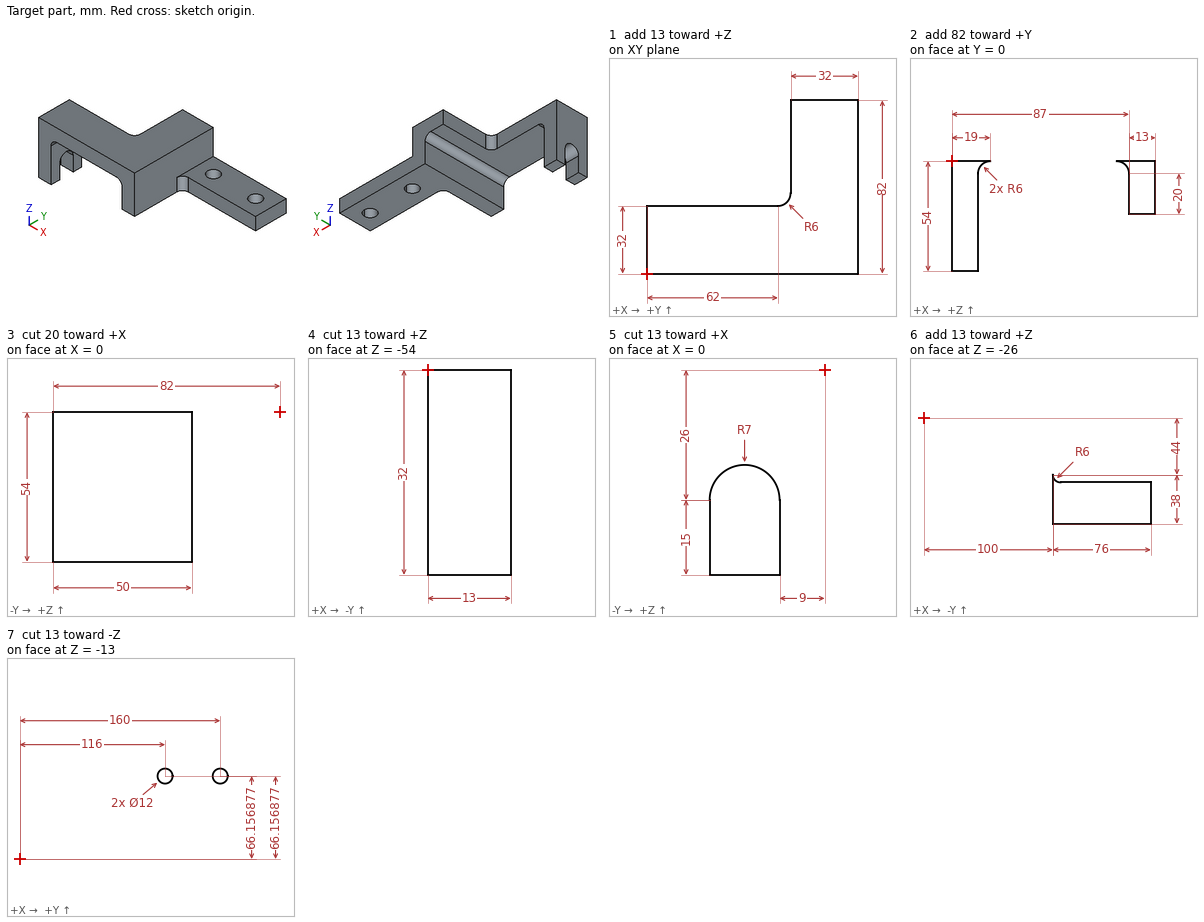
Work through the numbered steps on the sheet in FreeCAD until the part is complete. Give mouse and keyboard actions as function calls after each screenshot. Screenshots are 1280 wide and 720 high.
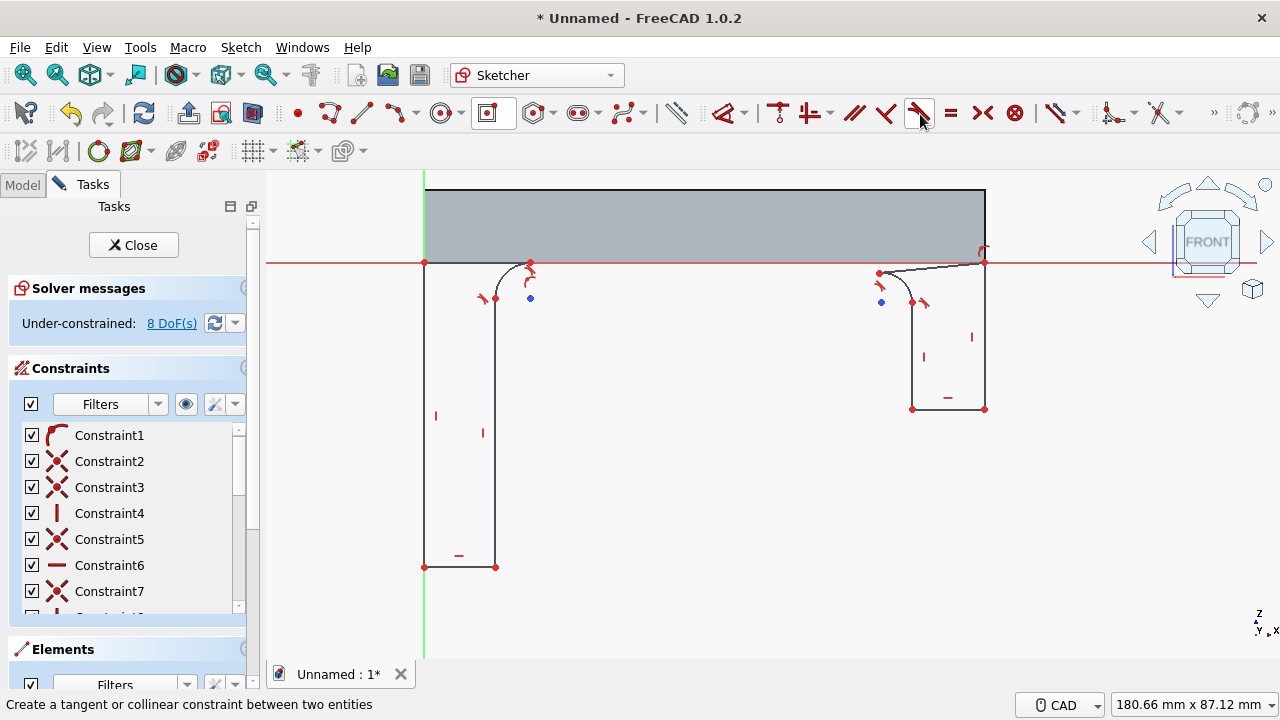
click(953, 266)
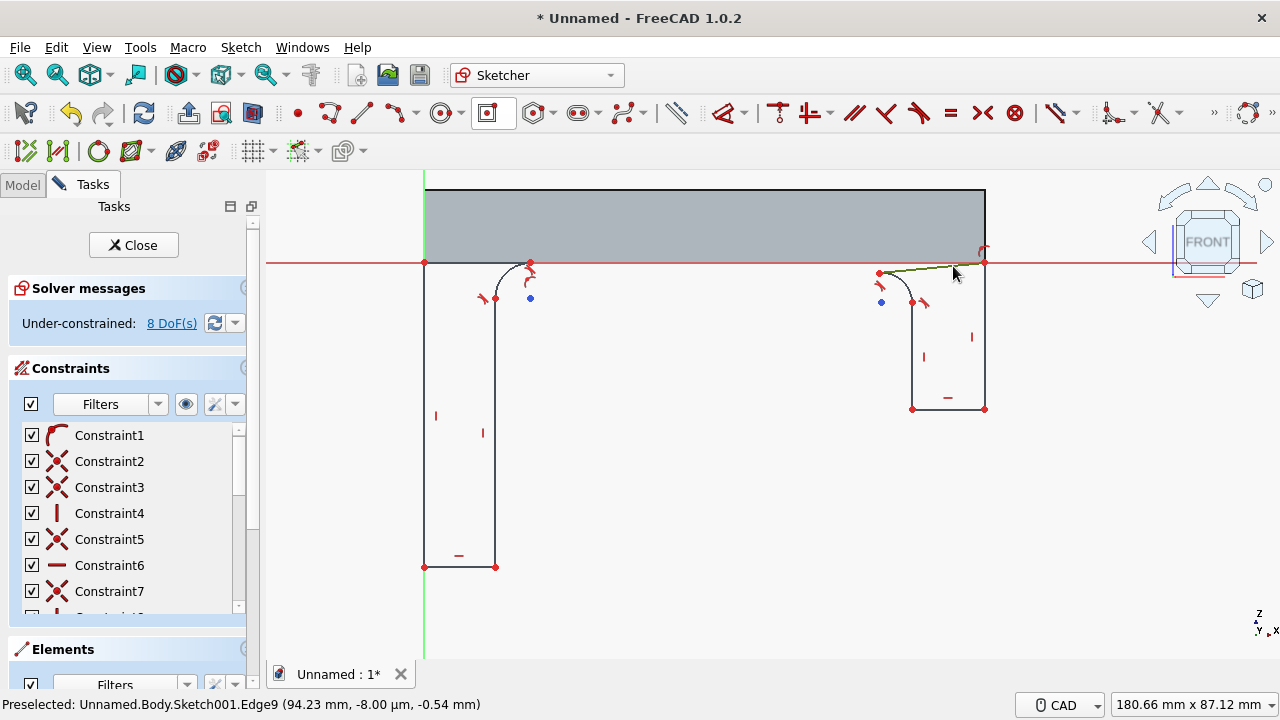
click(832, 114)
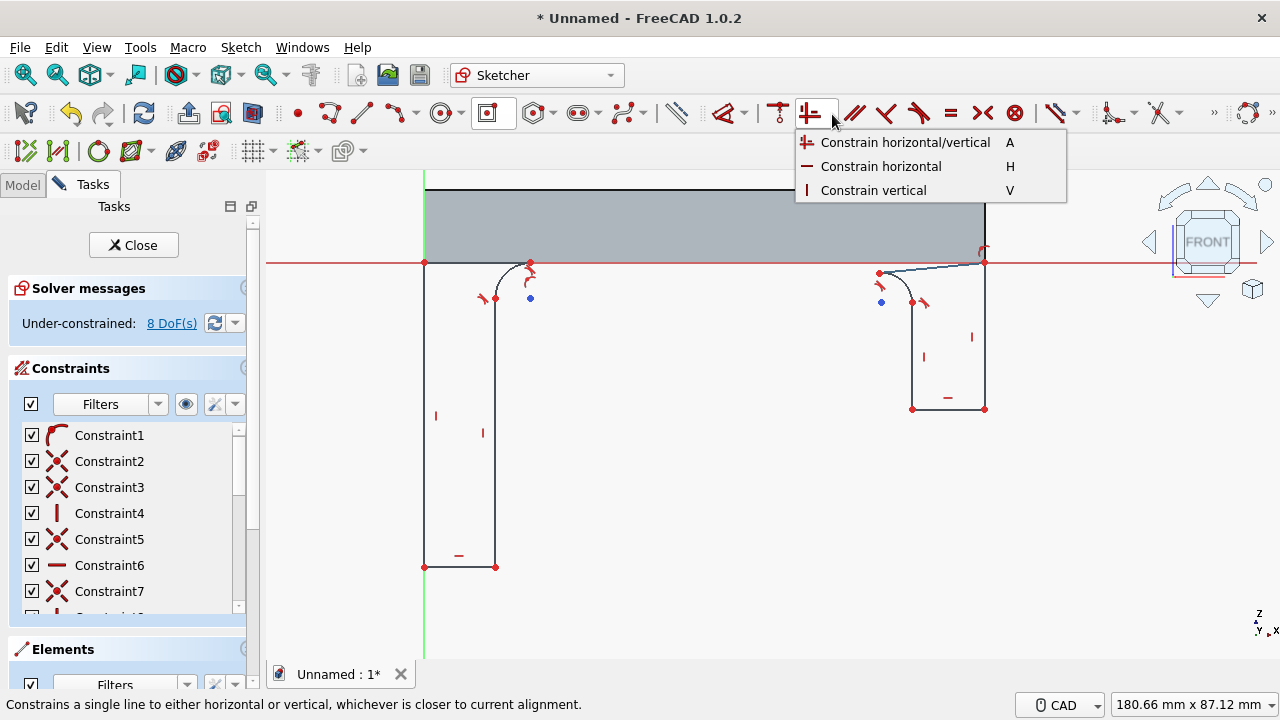
click(931, 166)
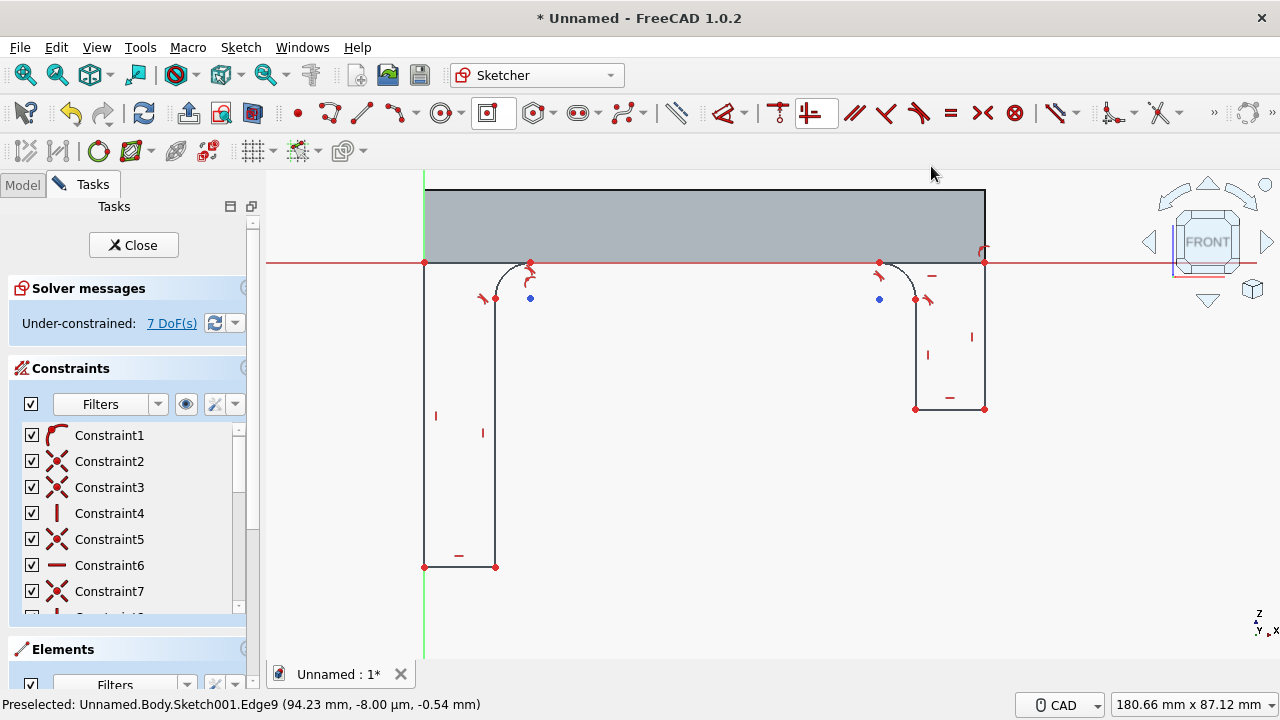
click(499, 282)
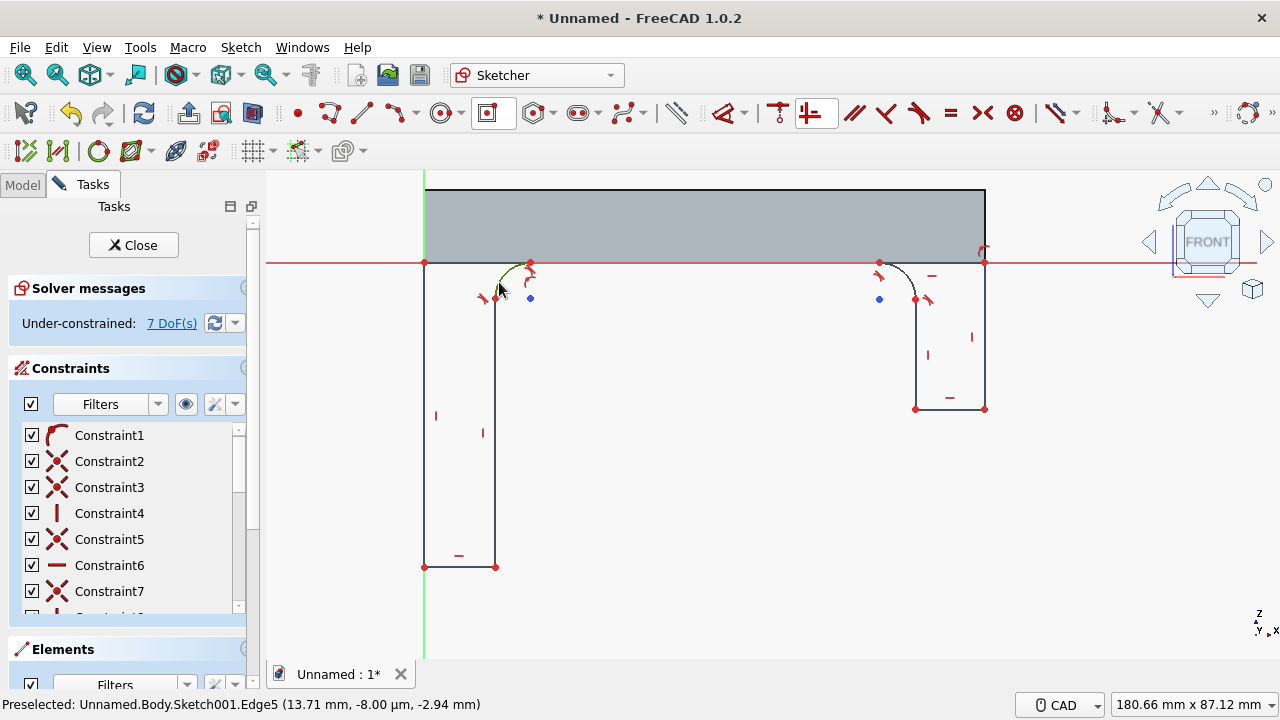
click(912, 283)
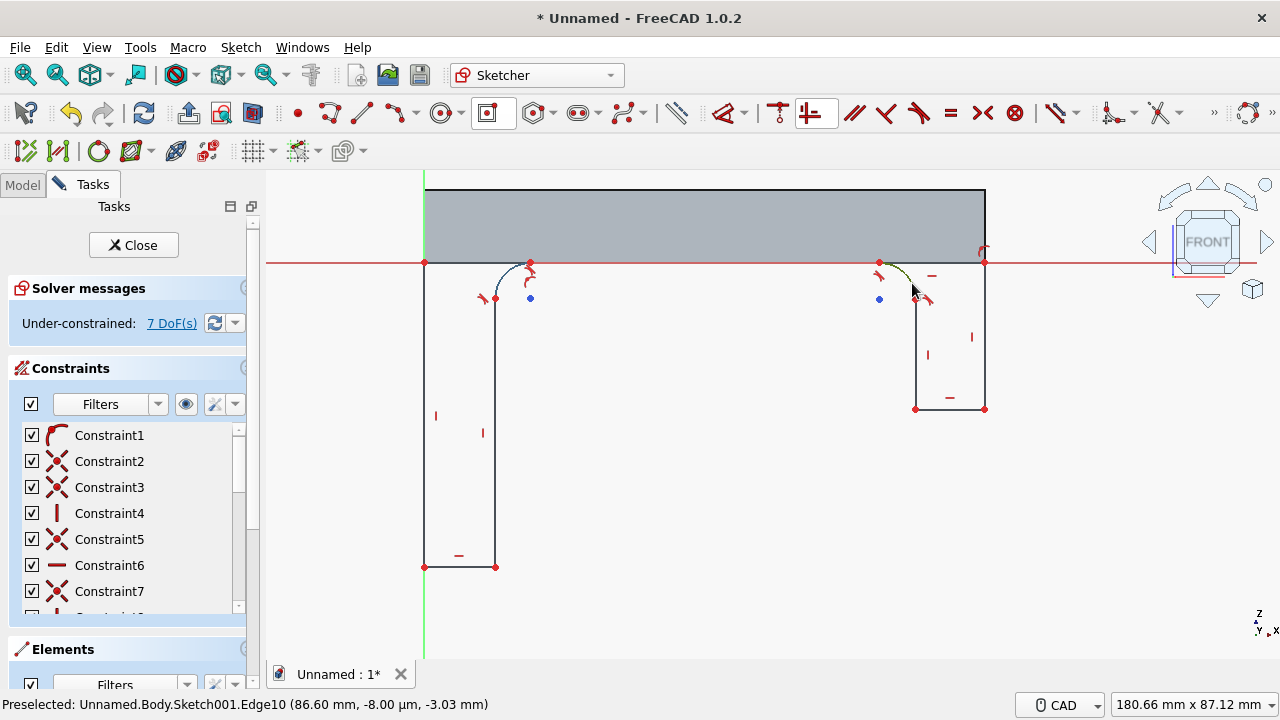
click(952, 114)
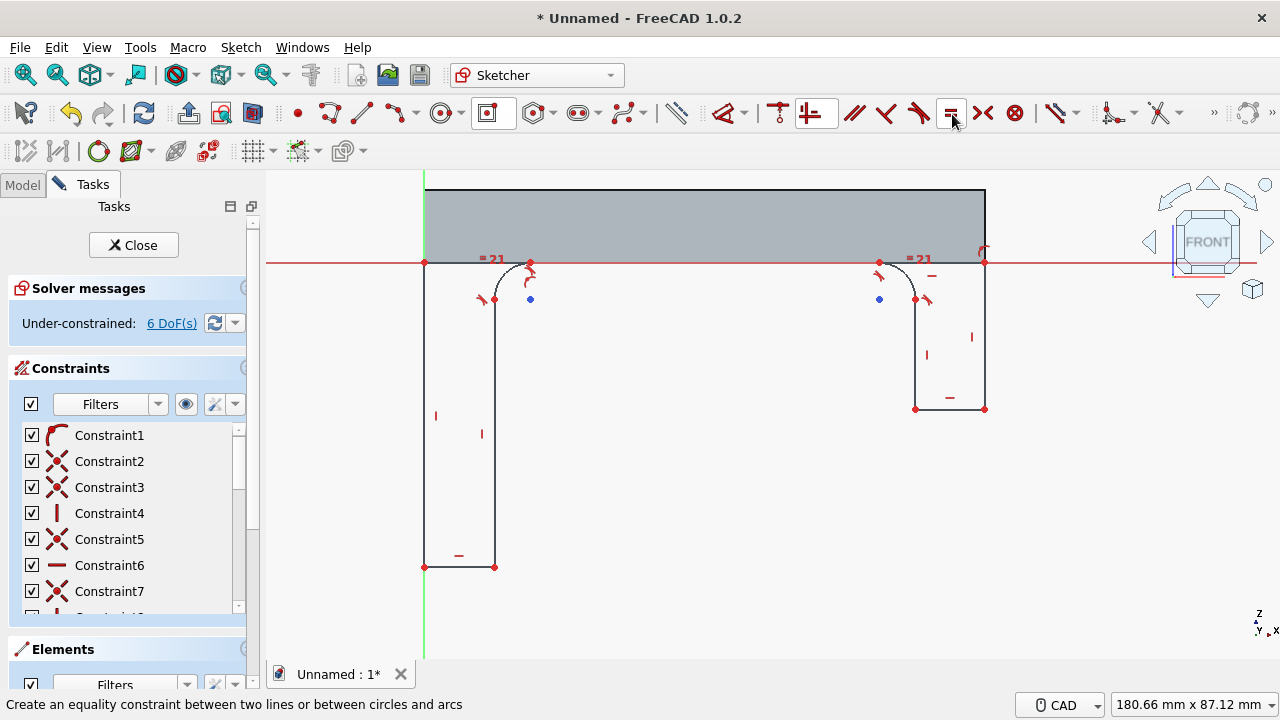
click(724, 114)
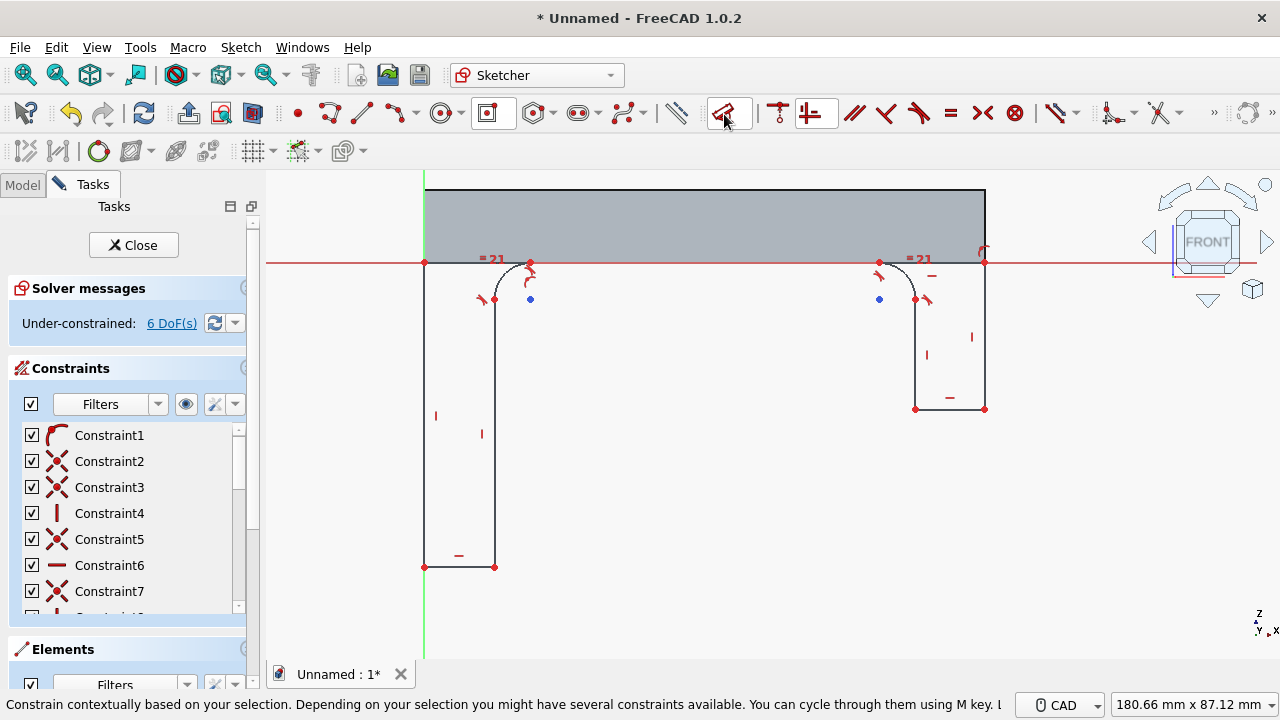
click(499, 283)
click(493, 243)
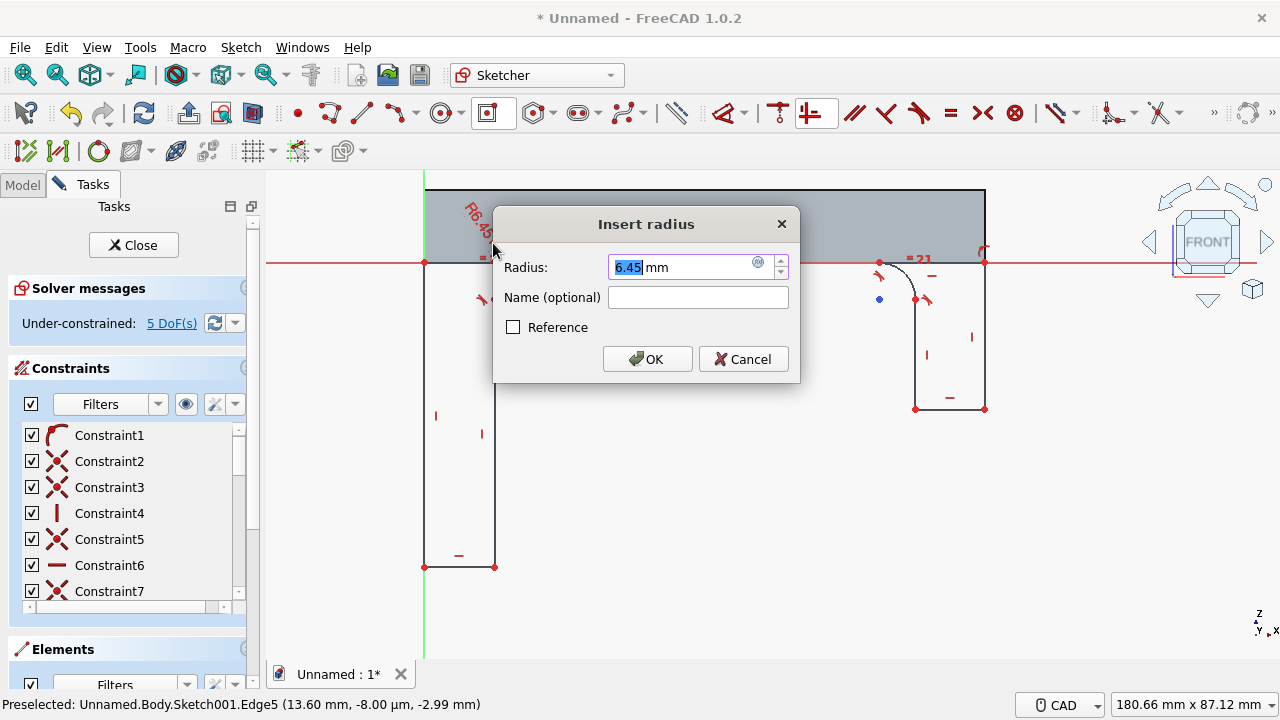
text(6)
key(Return)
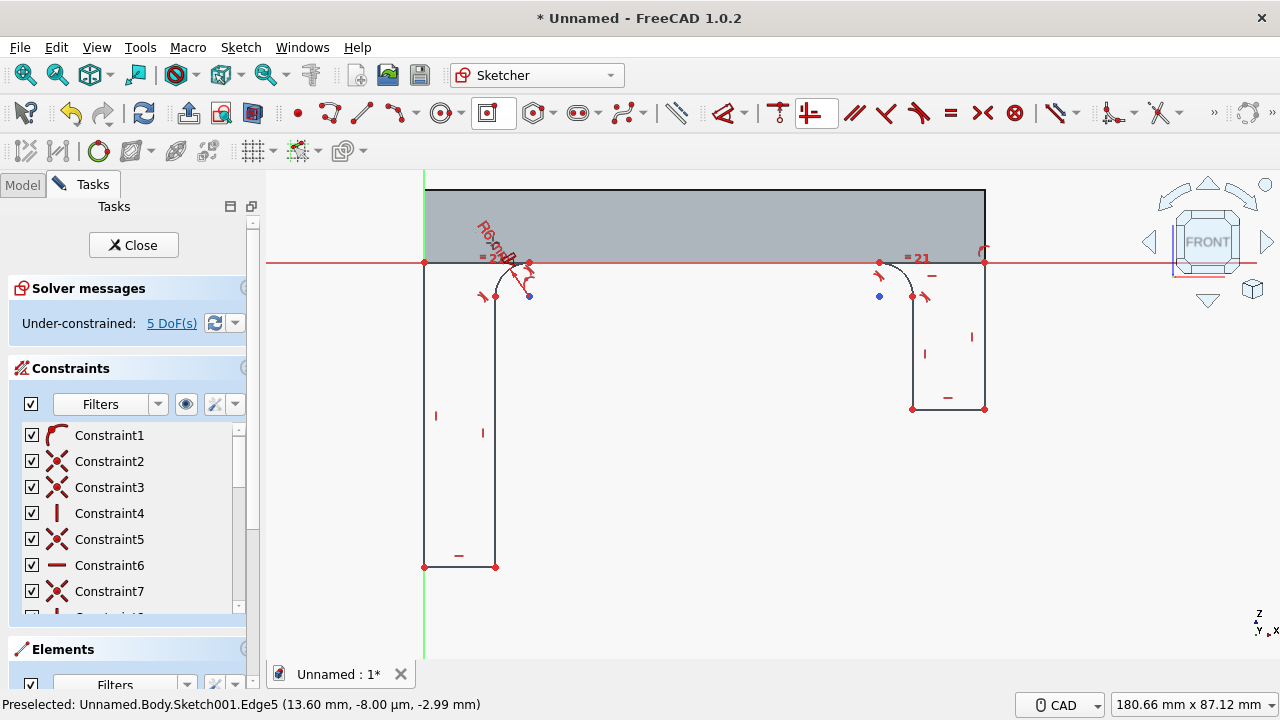
click(498, 263)
click(477, 297)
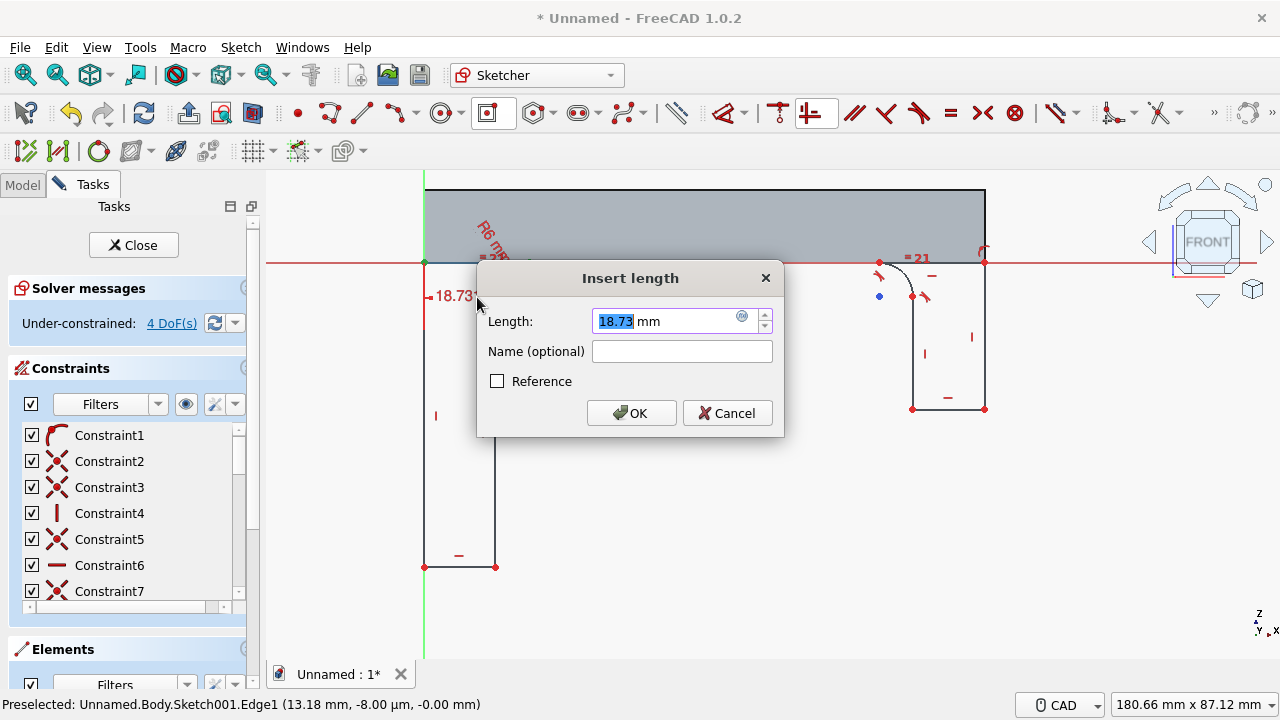
text(19)
key(Return)